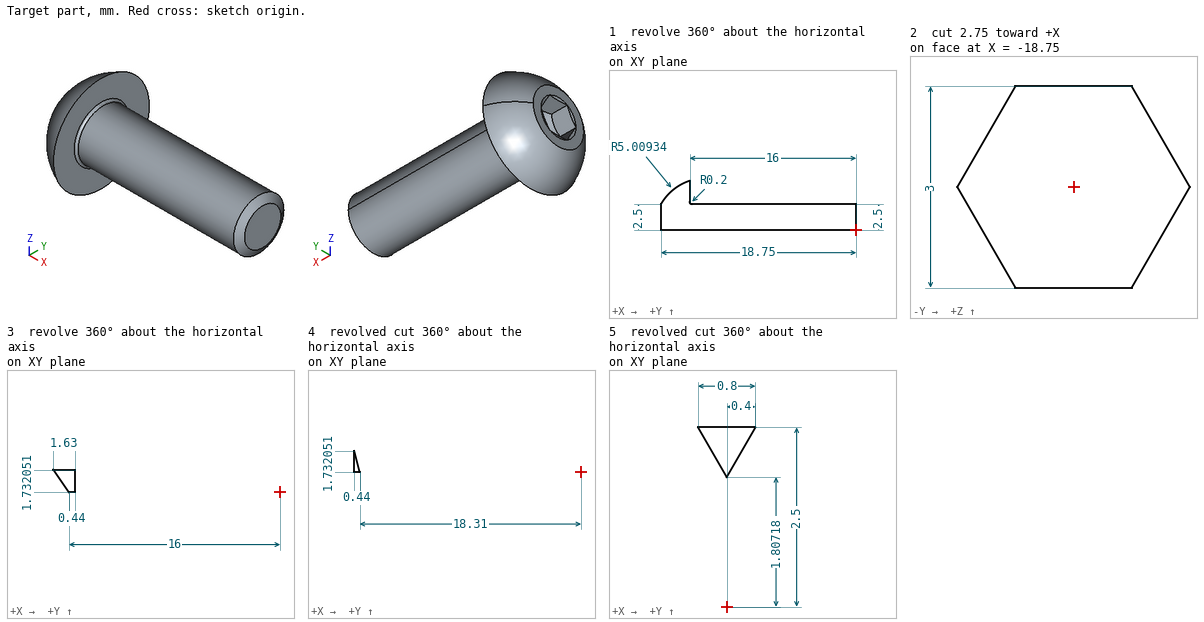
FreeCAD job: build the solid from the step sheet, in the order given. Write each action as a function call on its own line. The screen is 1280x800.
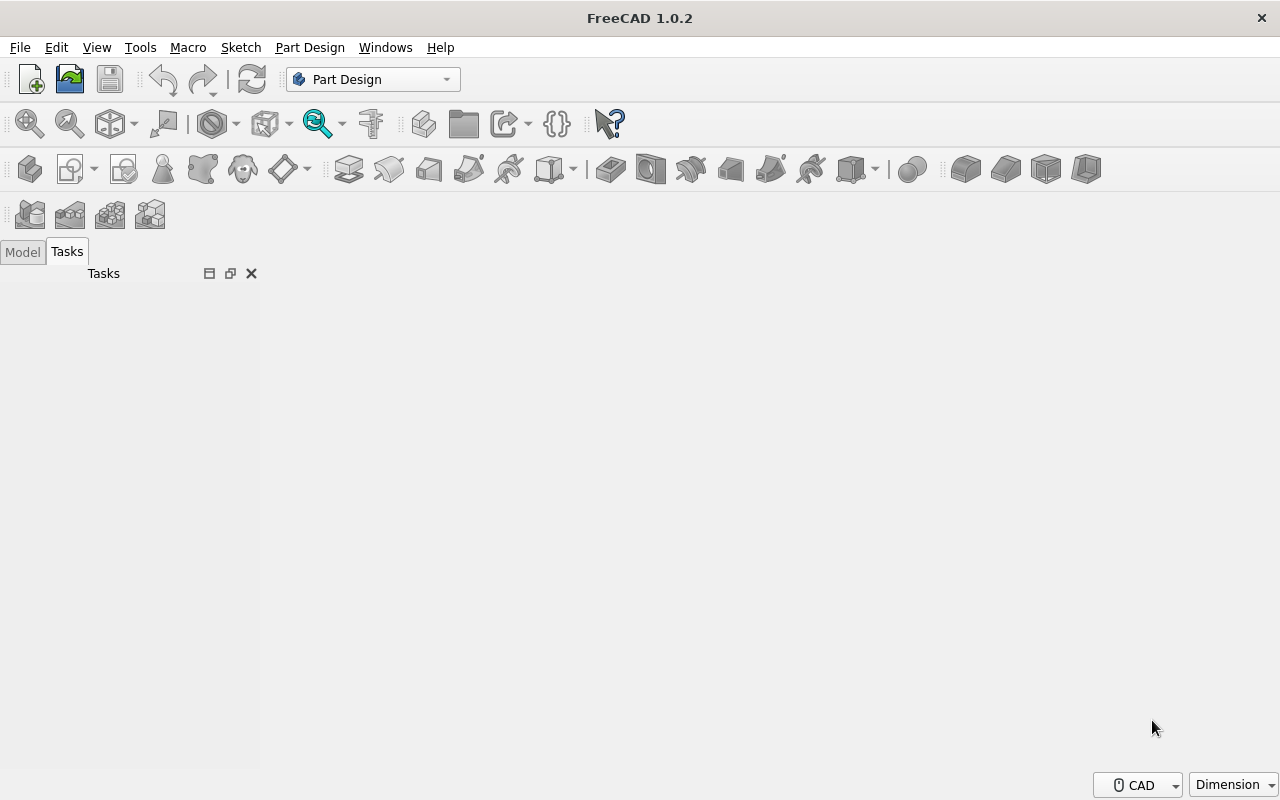
click(30, 80)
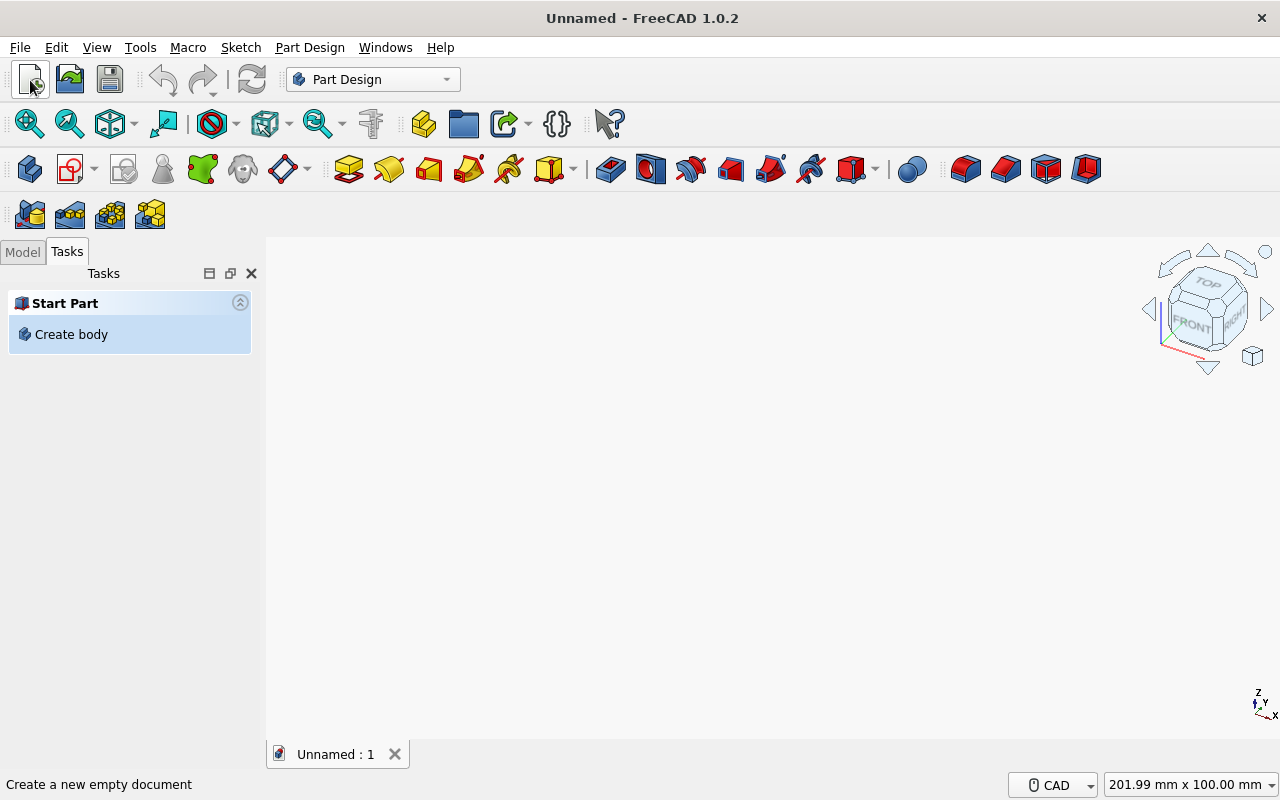
click(70, 170)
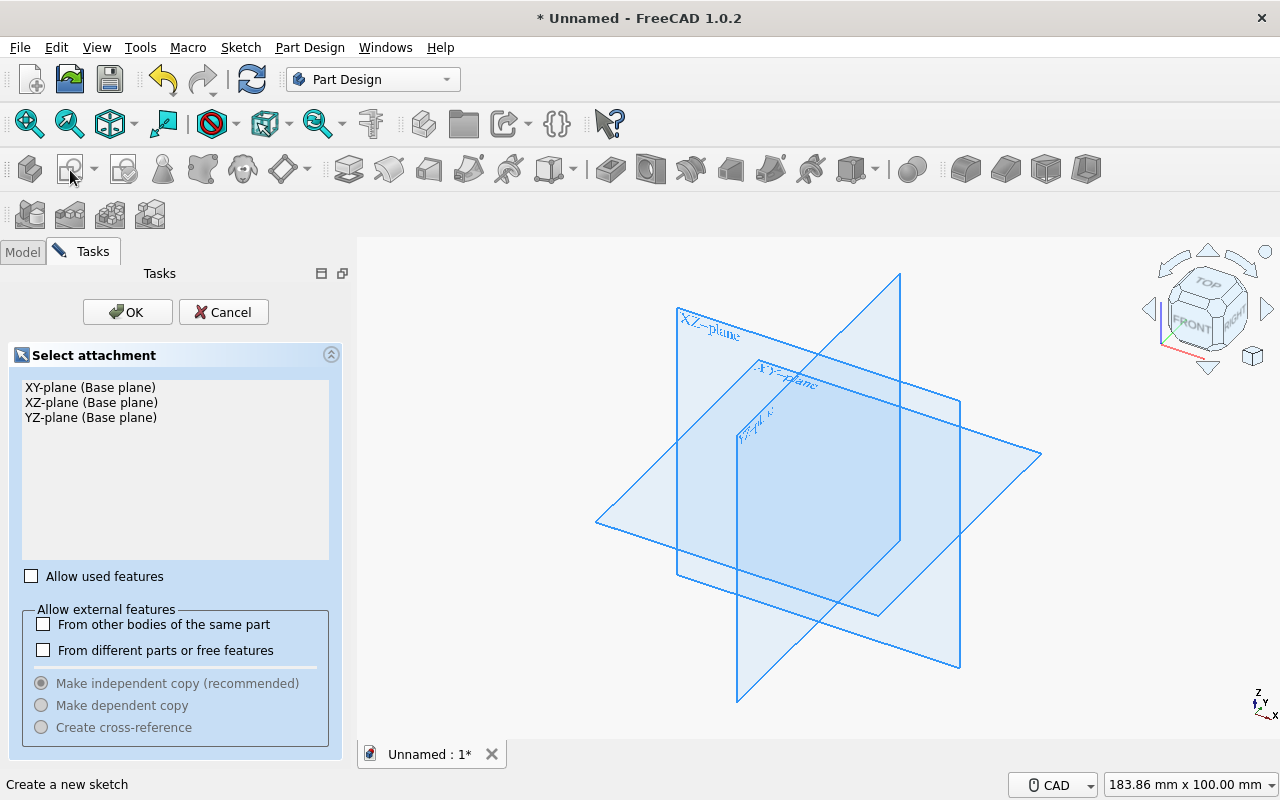
click(82, 388)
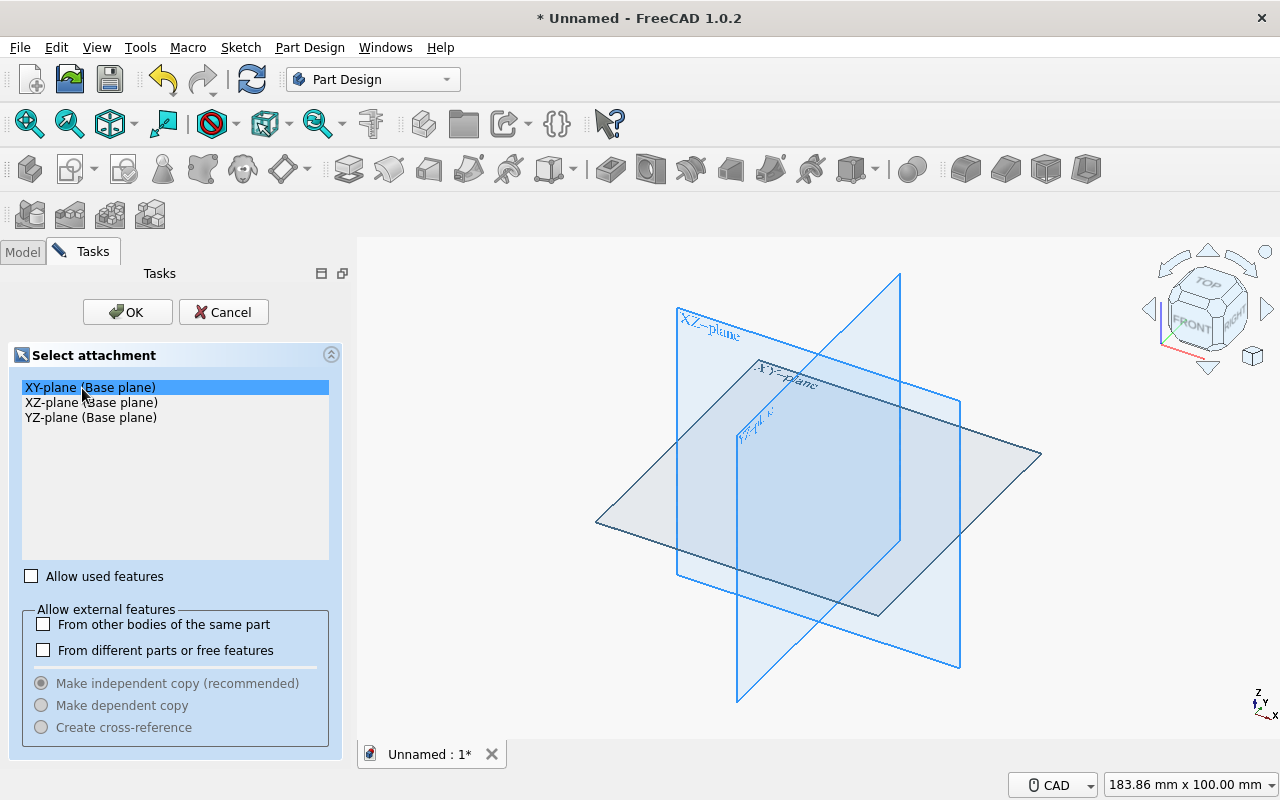
click(128, 312)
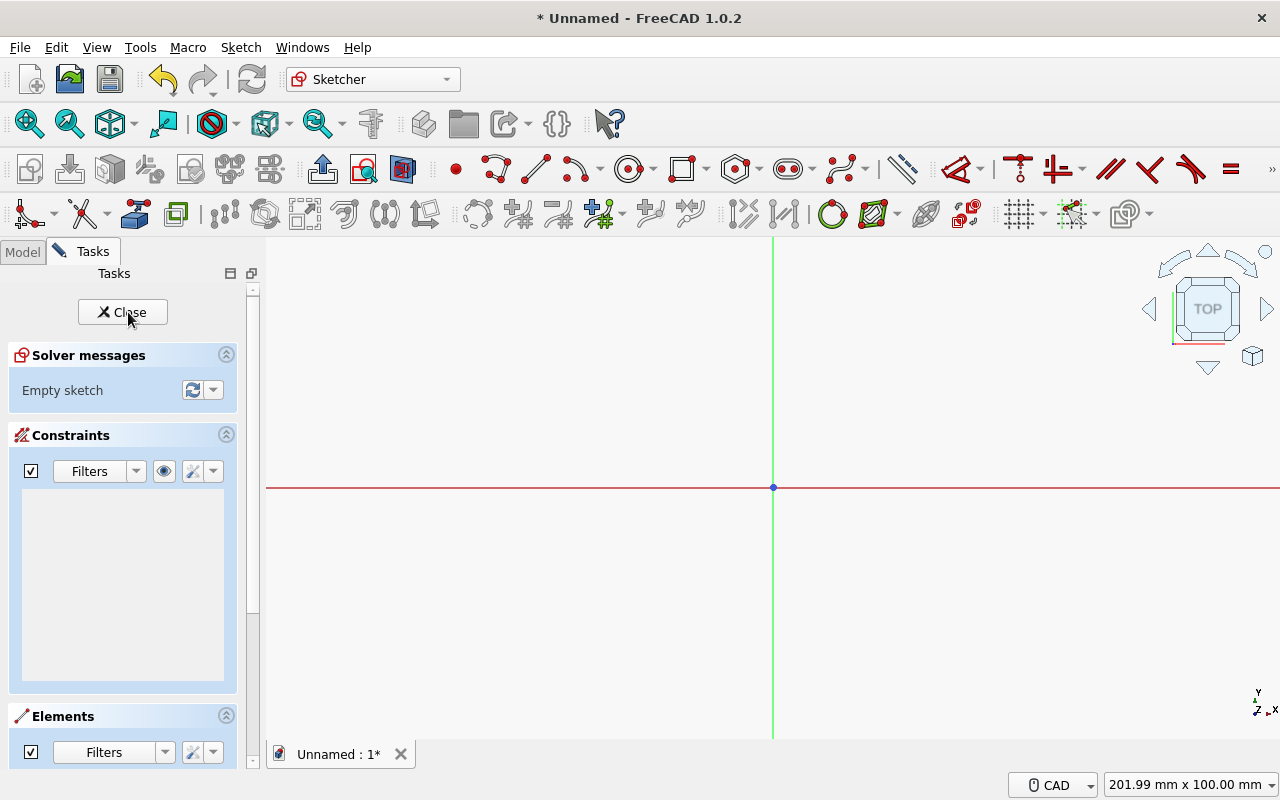
scroll(730, 474, up, 9)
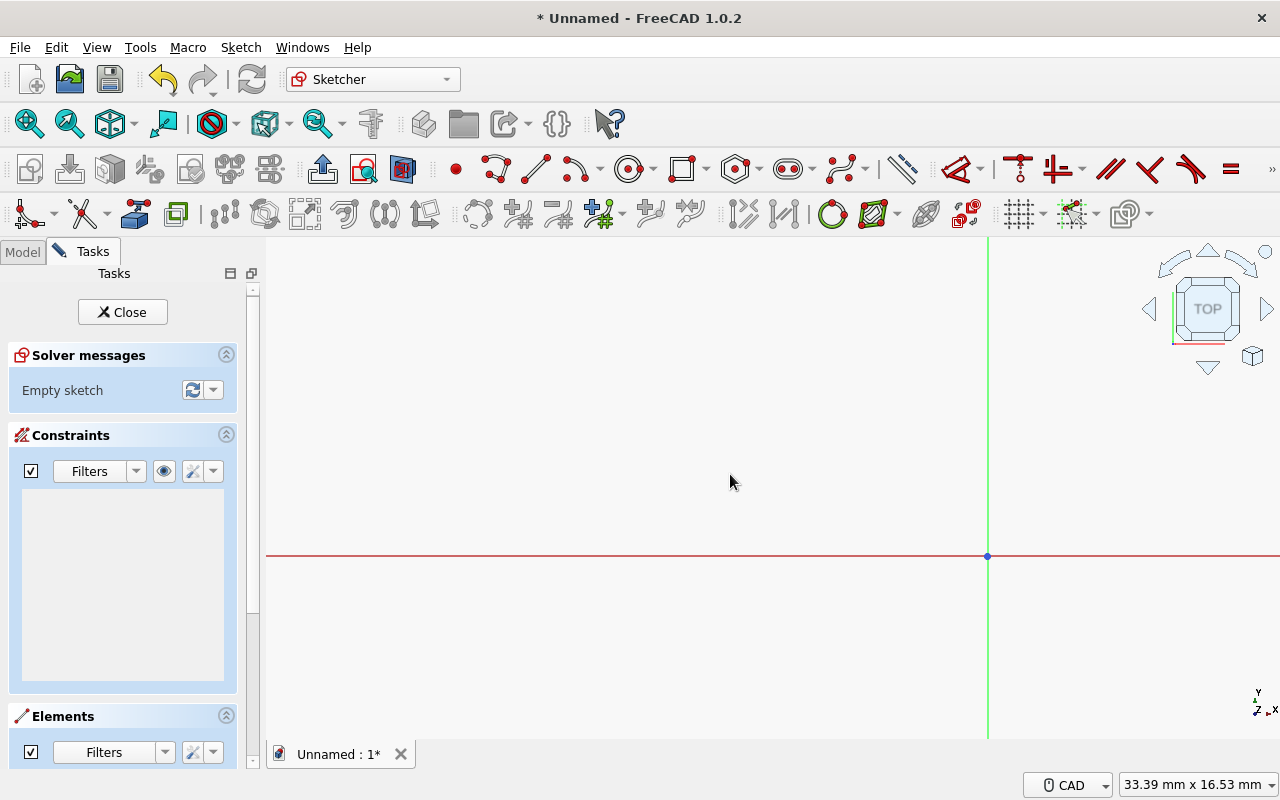
click(536, 170)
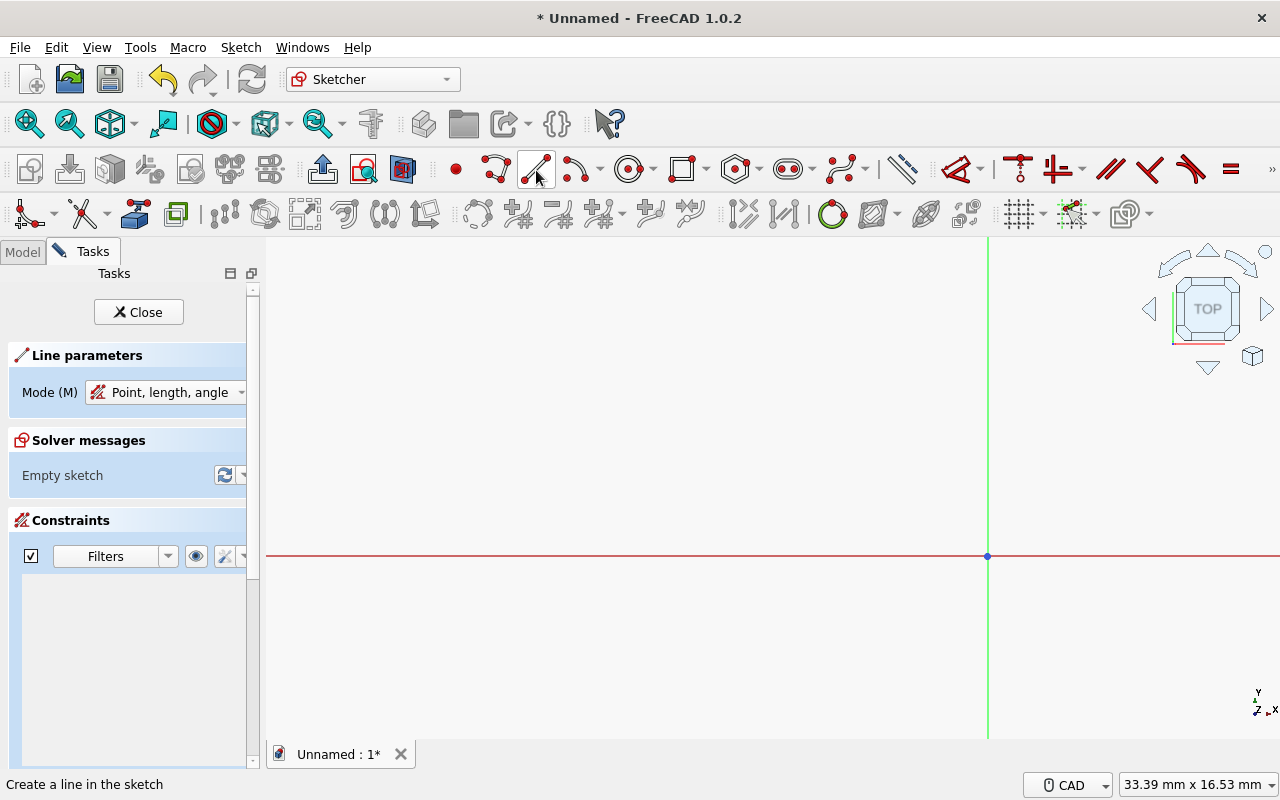
click(502, 474)
click(502, 412)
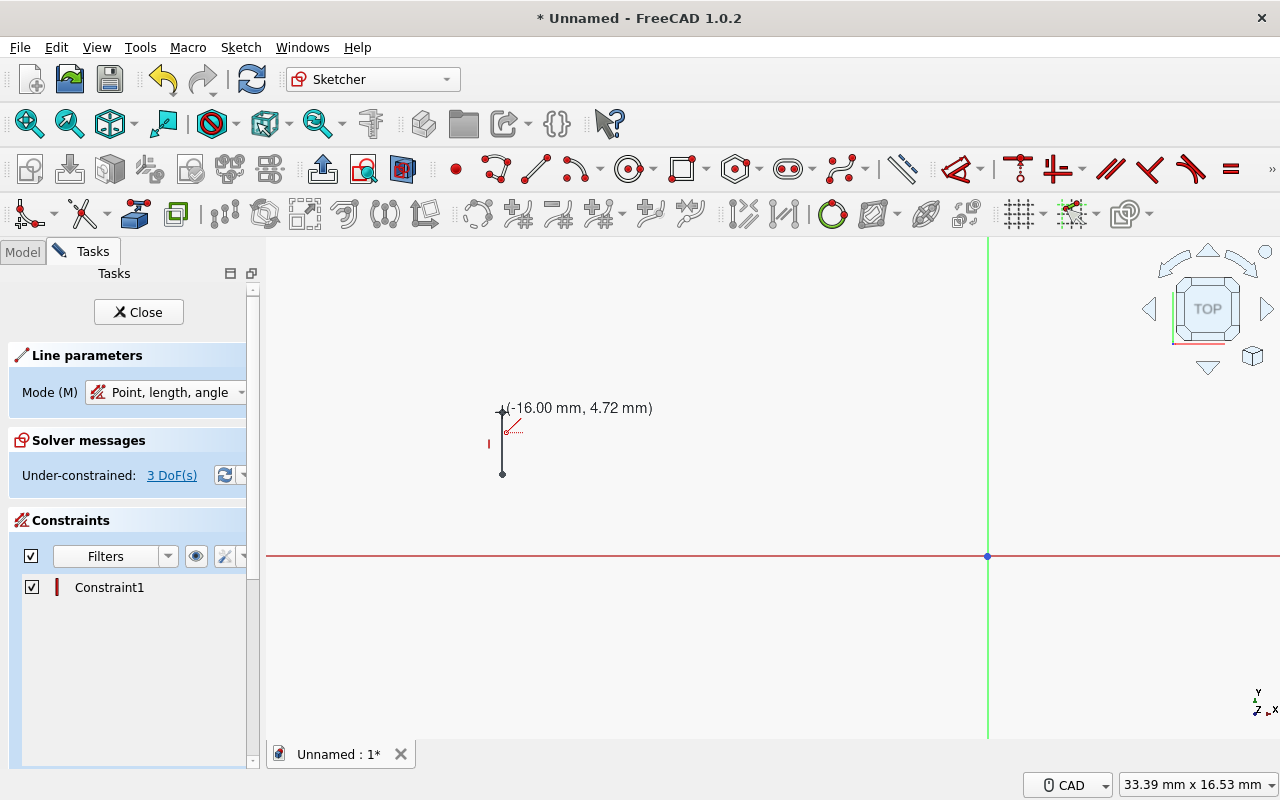
click(496, 170)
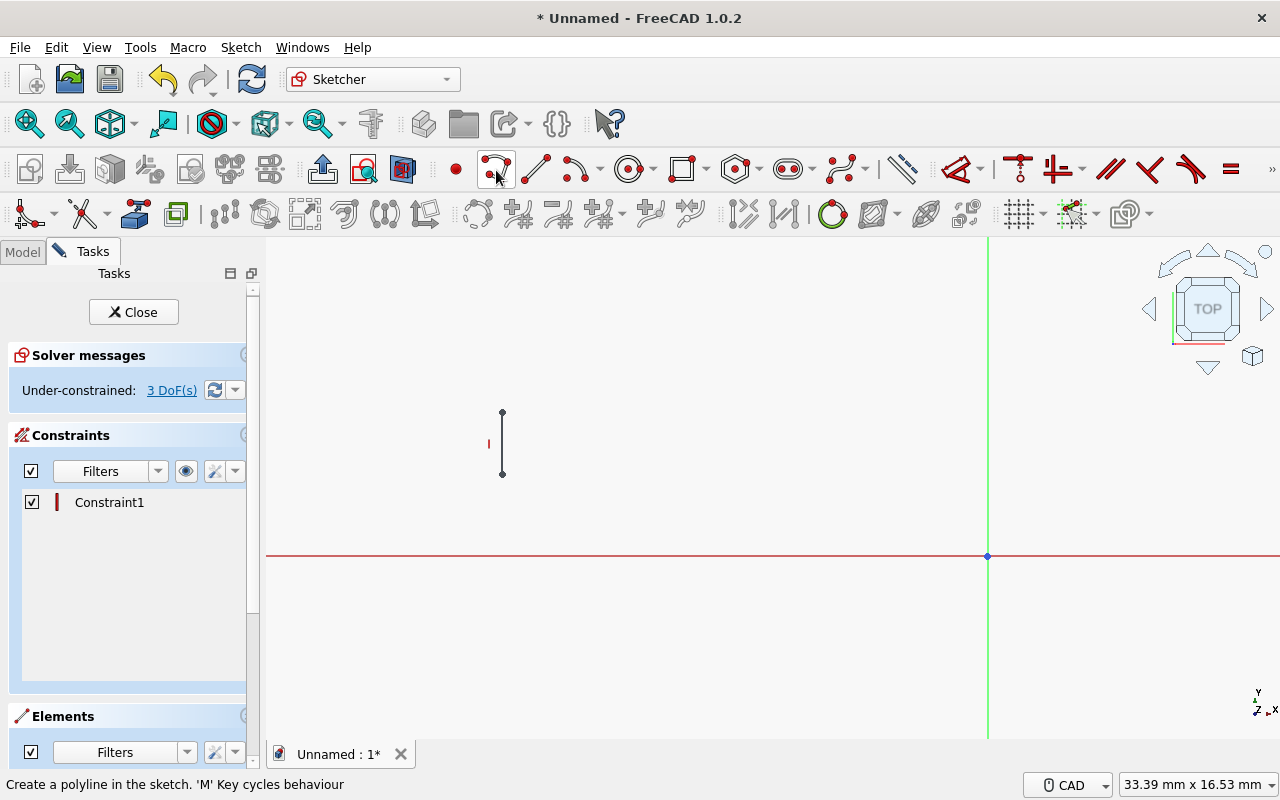
click(418, 480)
click(418, 556)
click(988, 556)
click(979, 480)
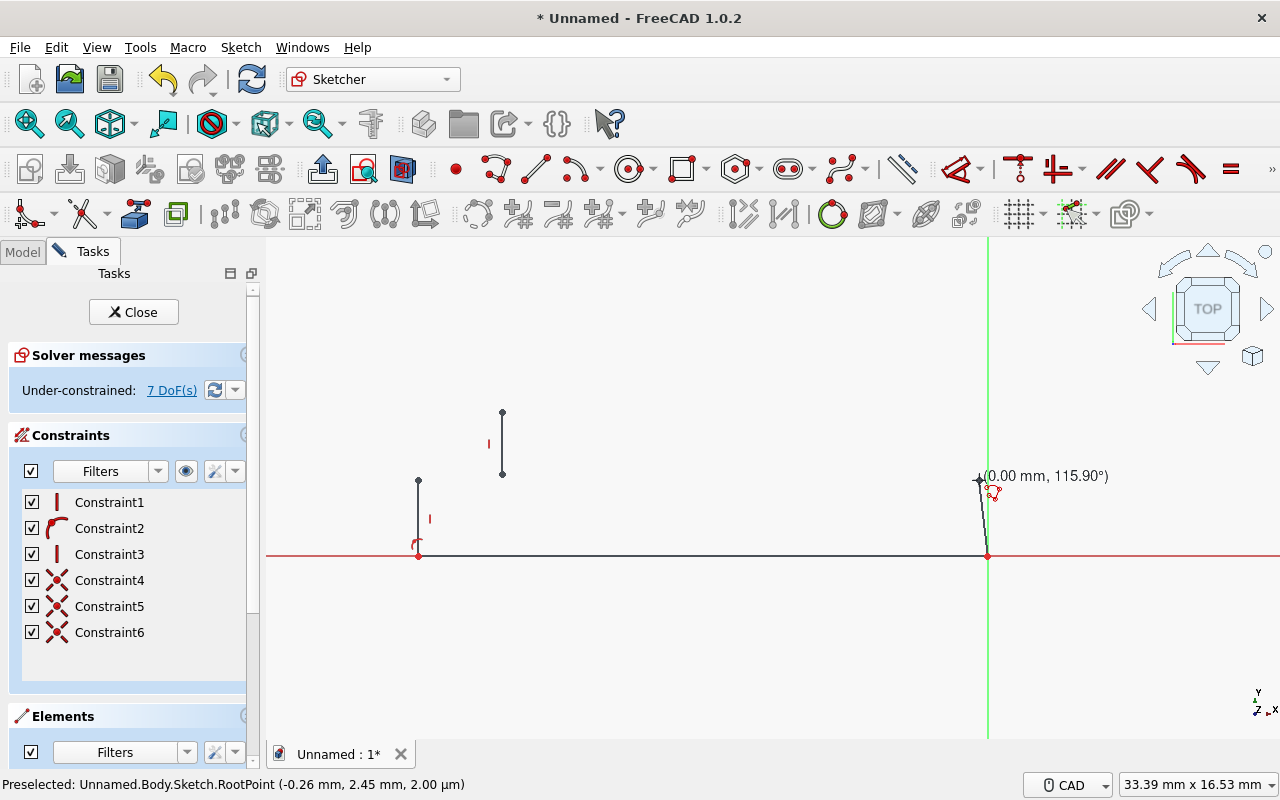
scroll(508, 480, up, 4)